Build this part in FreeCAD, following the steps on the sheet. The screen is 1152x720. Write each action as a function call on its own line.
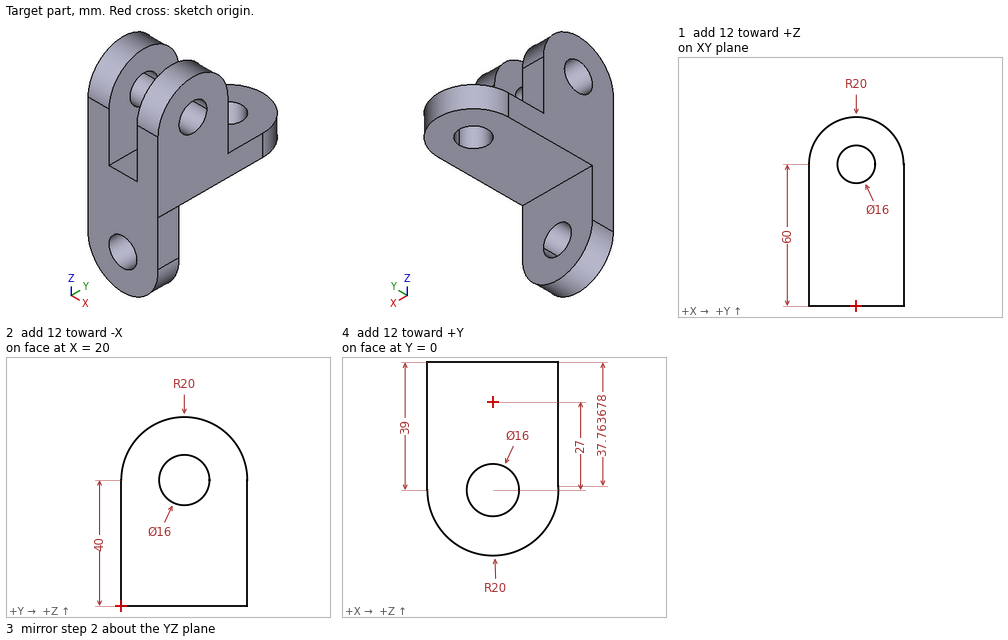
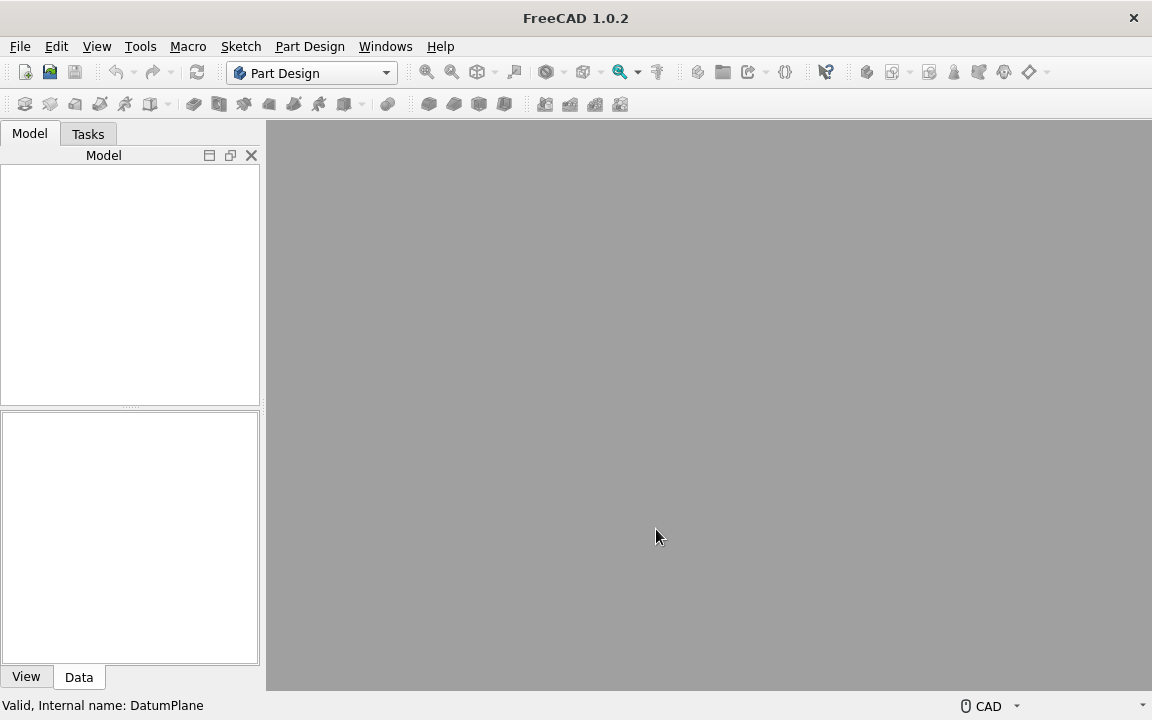
key(ctrl+n)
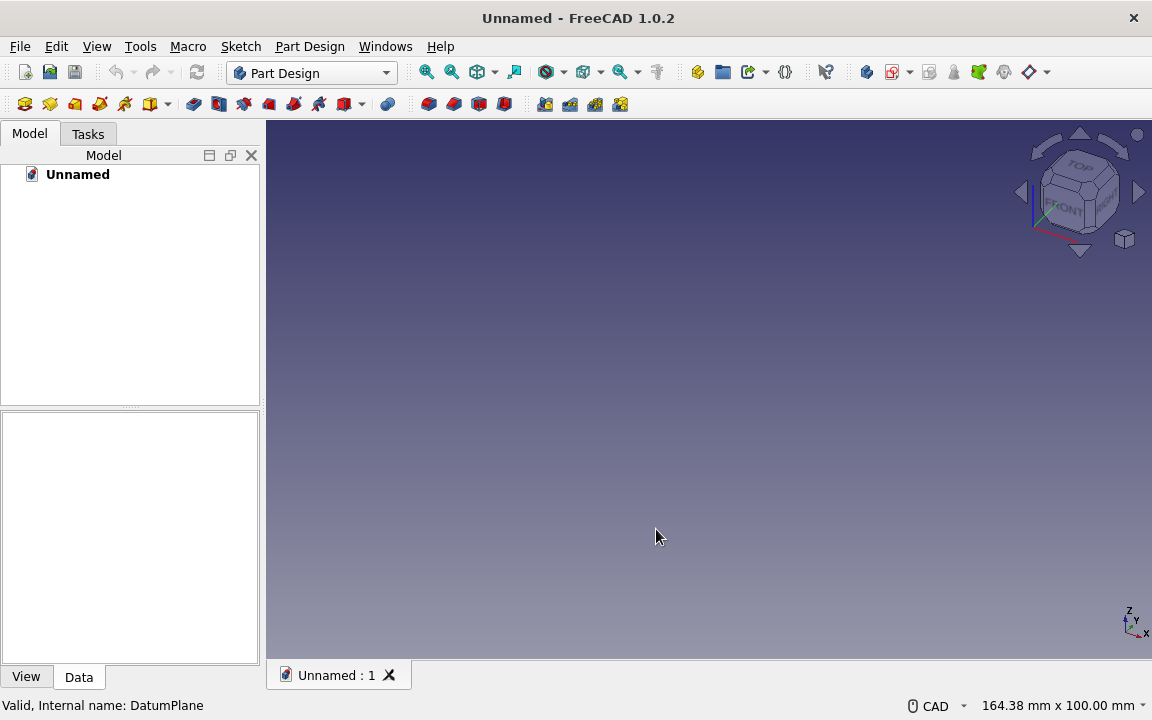
click(892, 72)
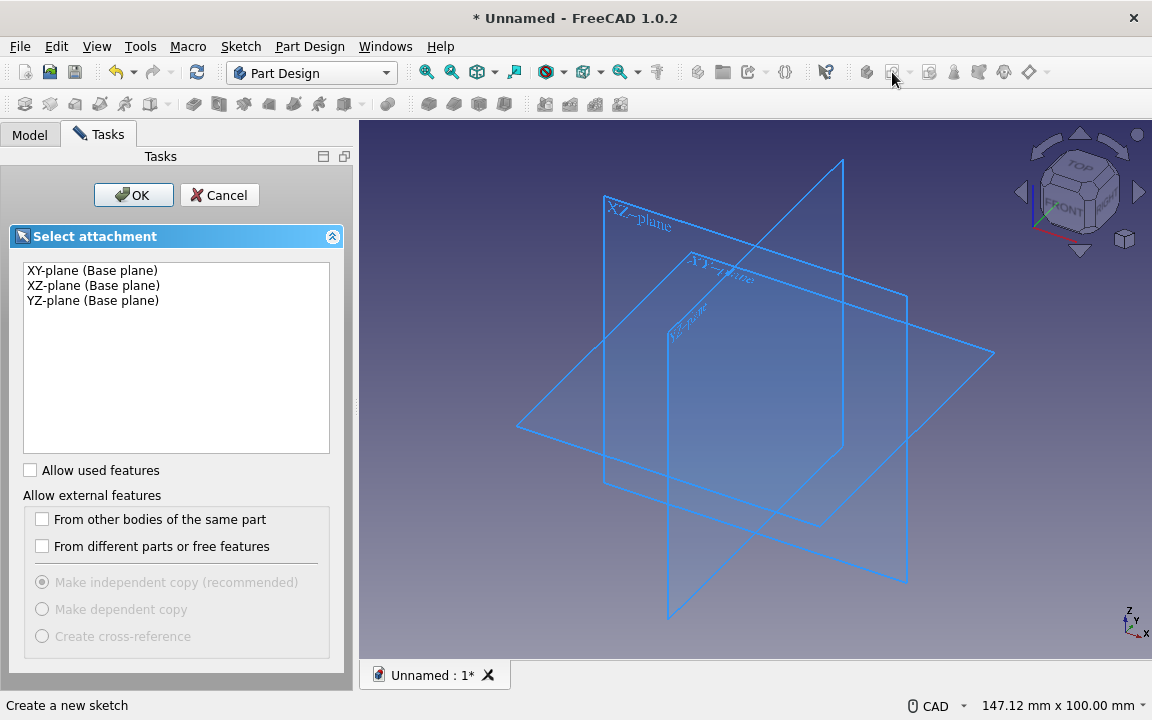
click(84, 270)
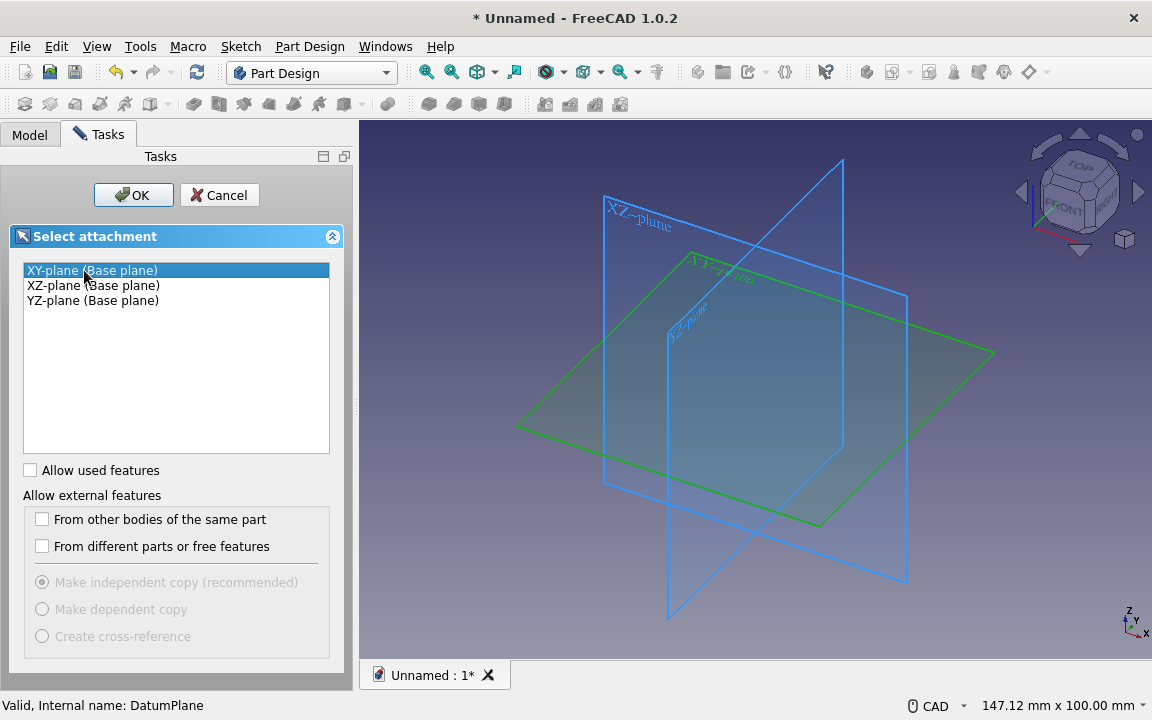
click(134, 195)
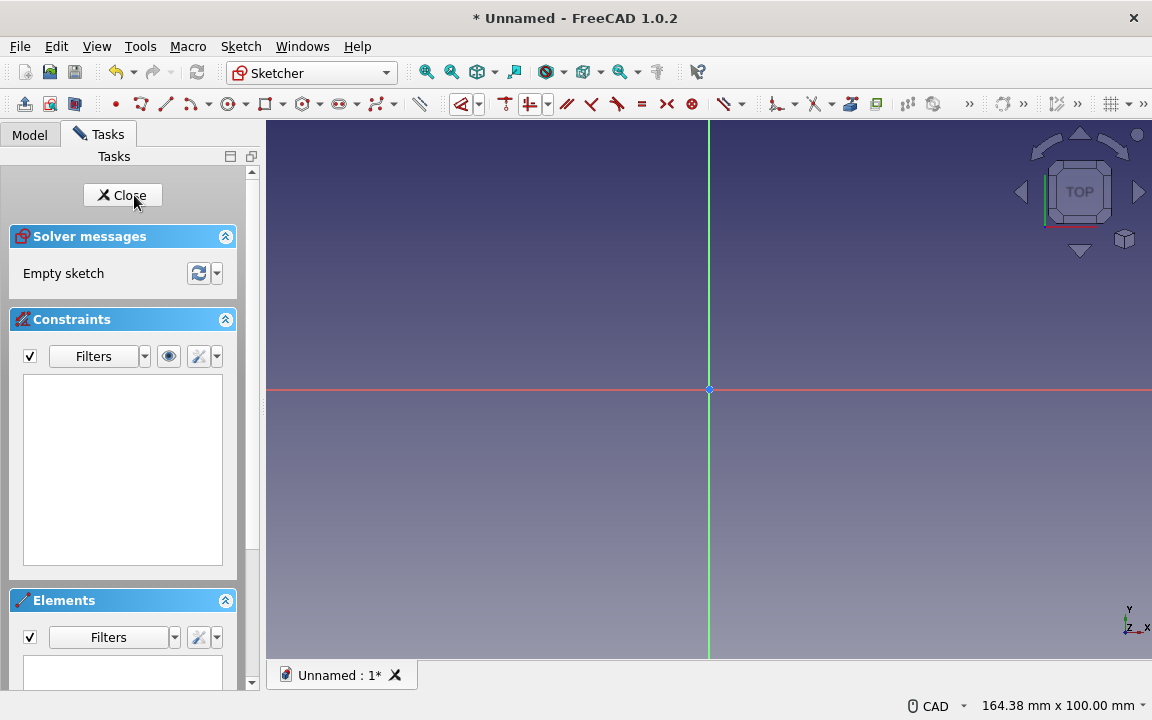
scroll(501, 631, down, 2)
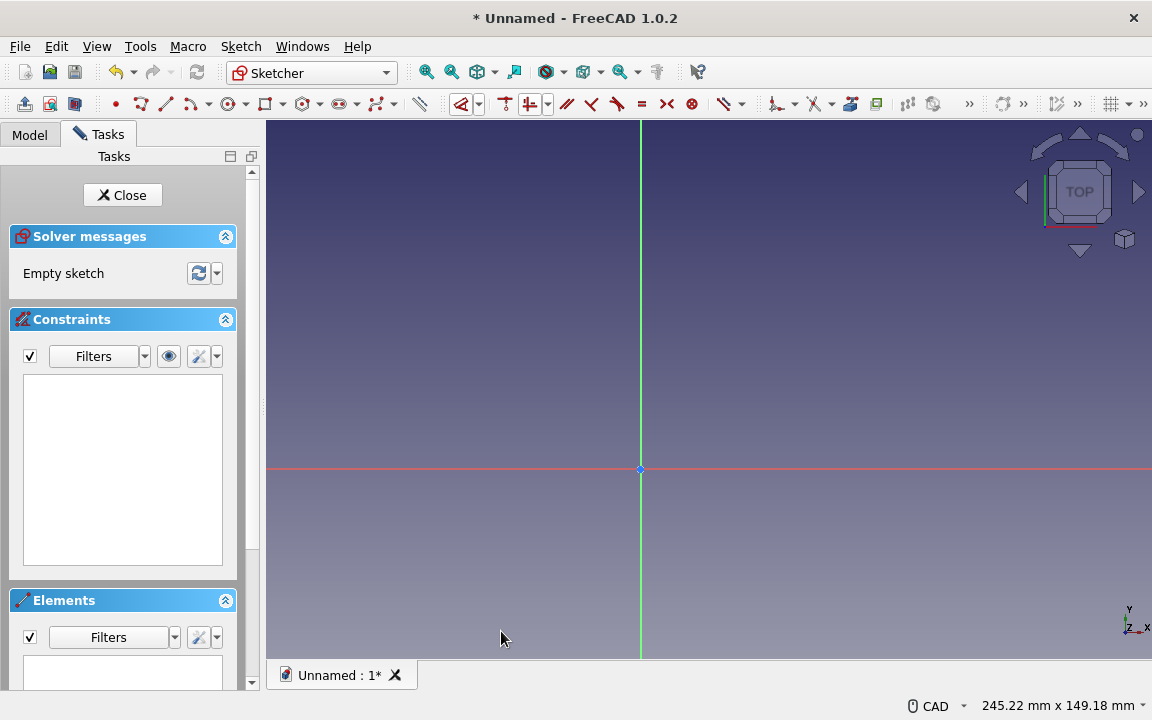
key(g)
key(m)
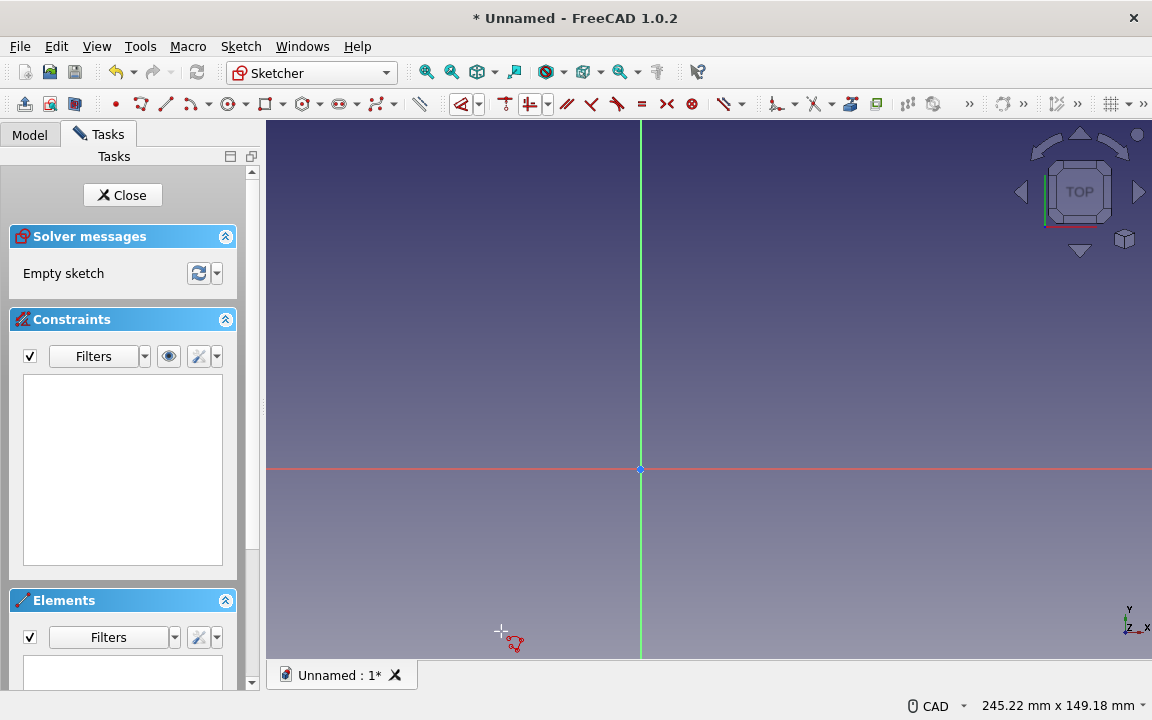
click(568, 253)
click(568, 469)
click(713, 460)
click(713, 253)
right_click(713, 253)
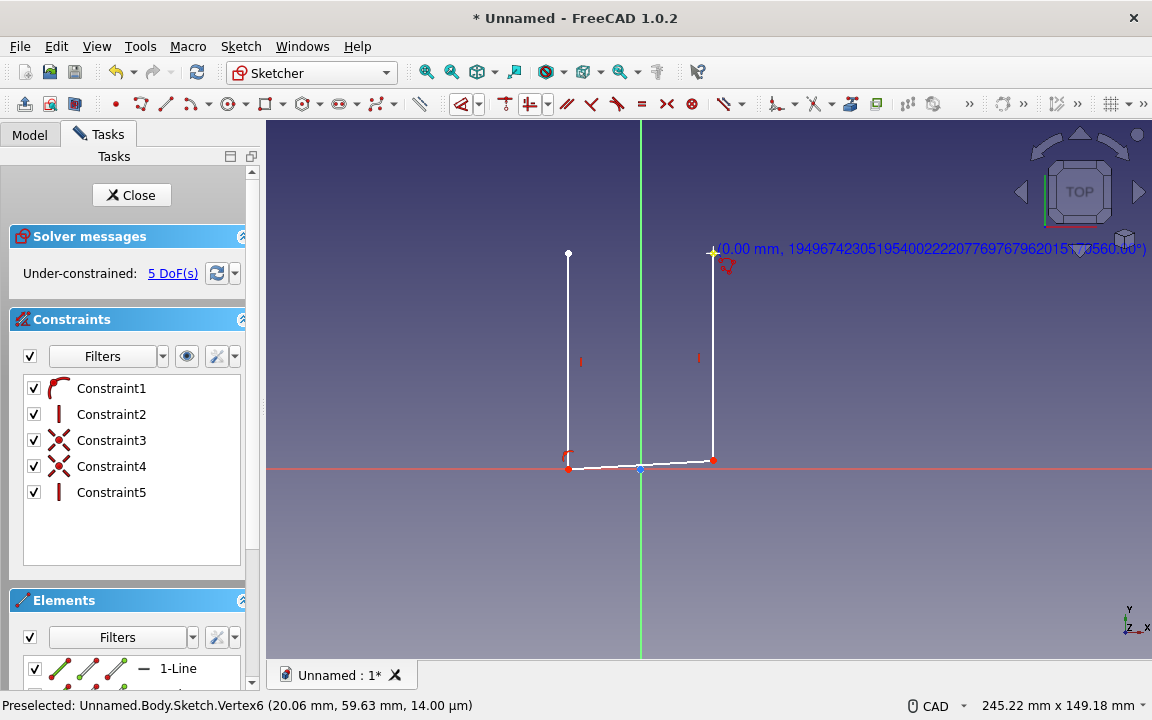
key(g)
key(3)
key(a)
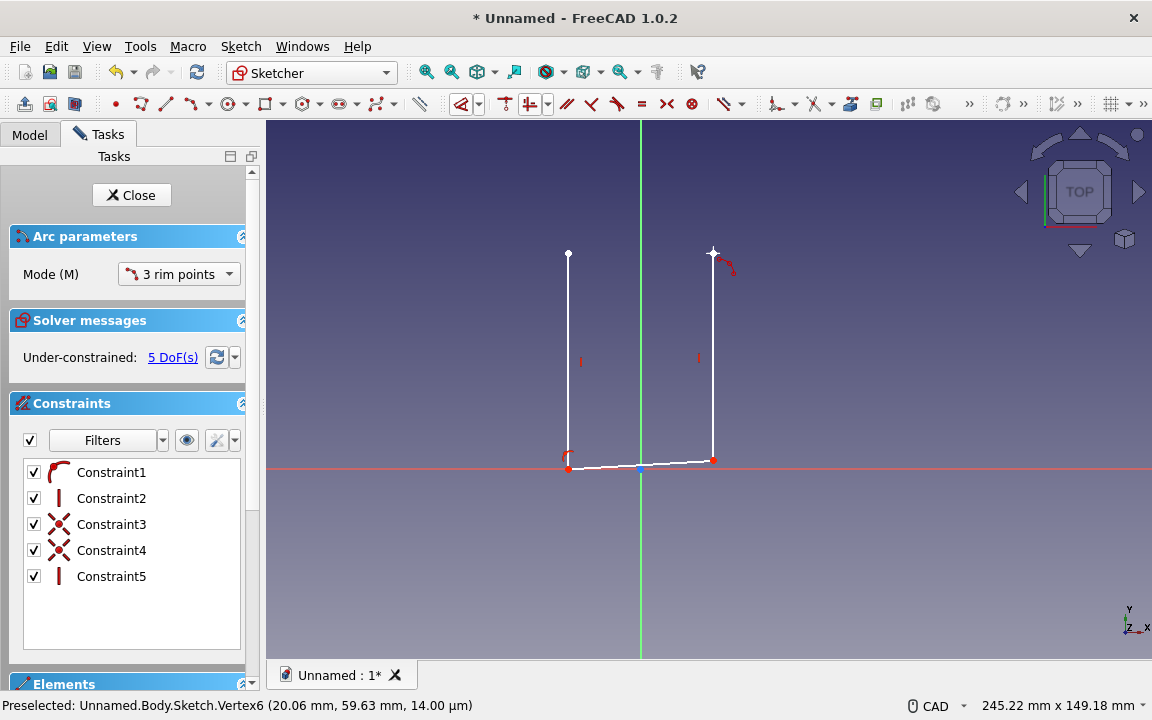
click(713, 254)
click(568, 254)
click(663, 184)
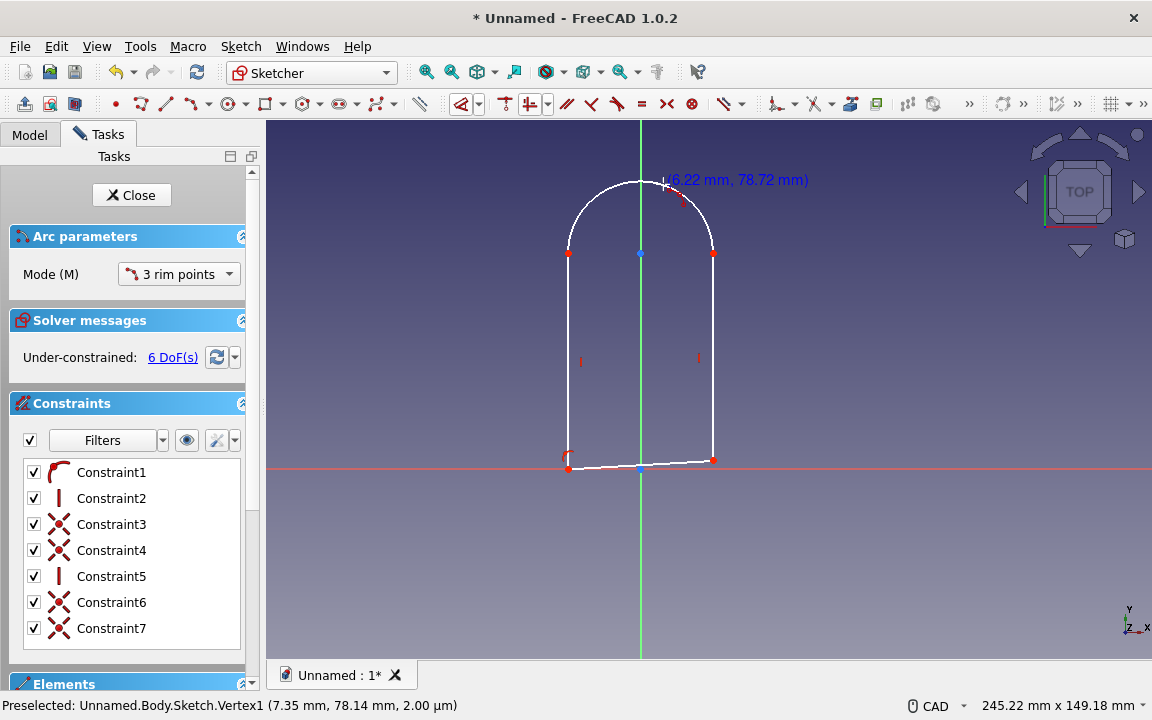
key(g)
key(c)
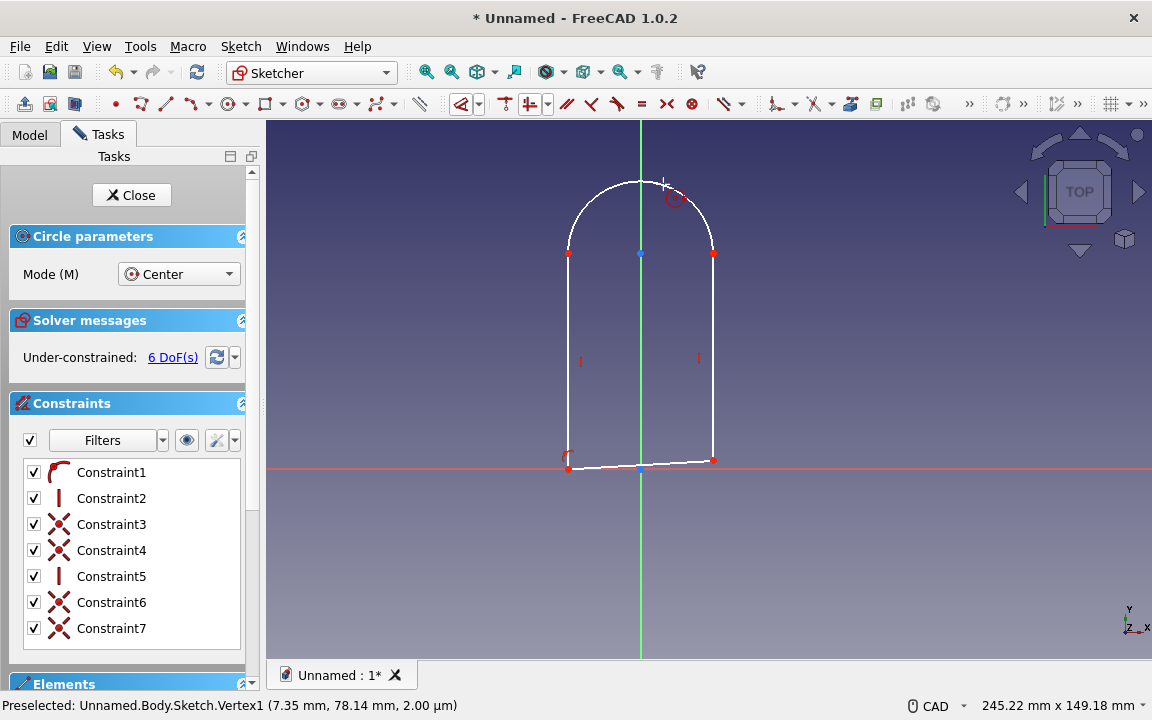
click(641, 253)
move(661, 232)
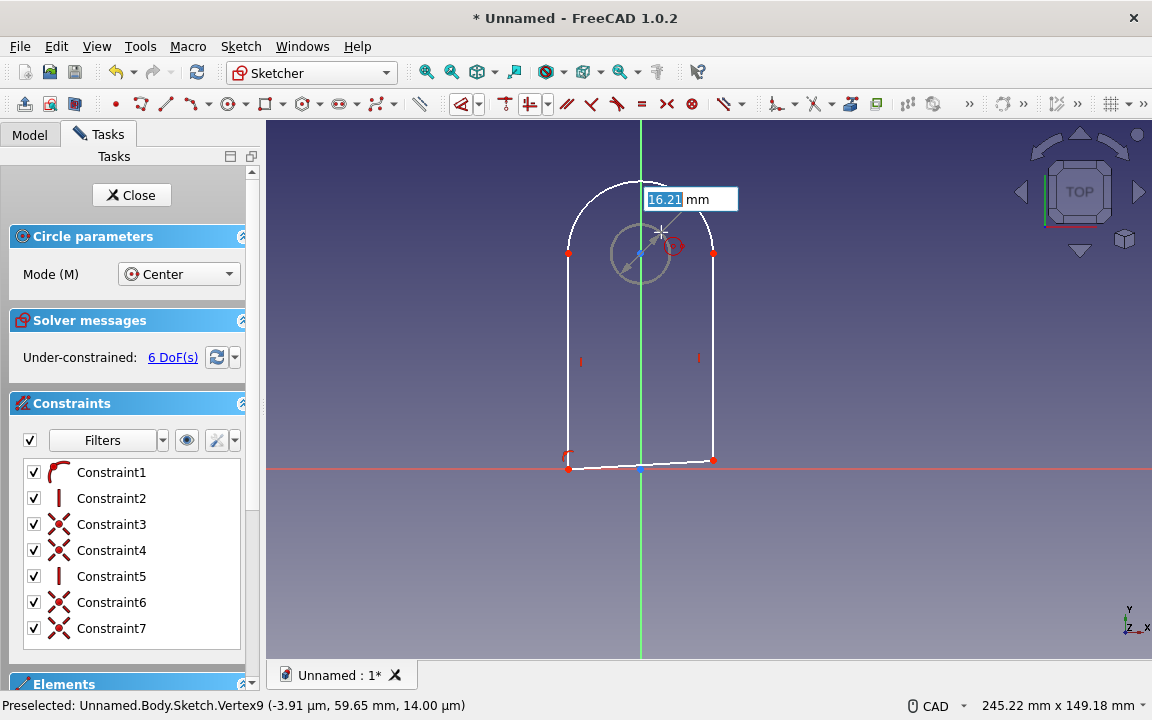
text(16)
key(Return)
key(Escape)